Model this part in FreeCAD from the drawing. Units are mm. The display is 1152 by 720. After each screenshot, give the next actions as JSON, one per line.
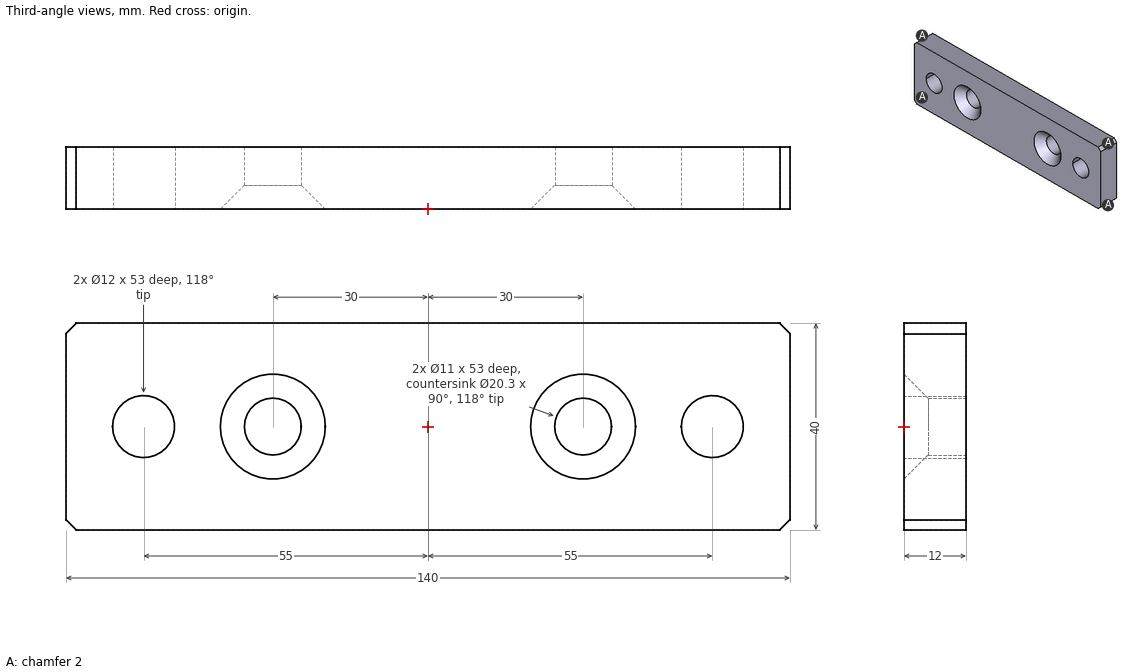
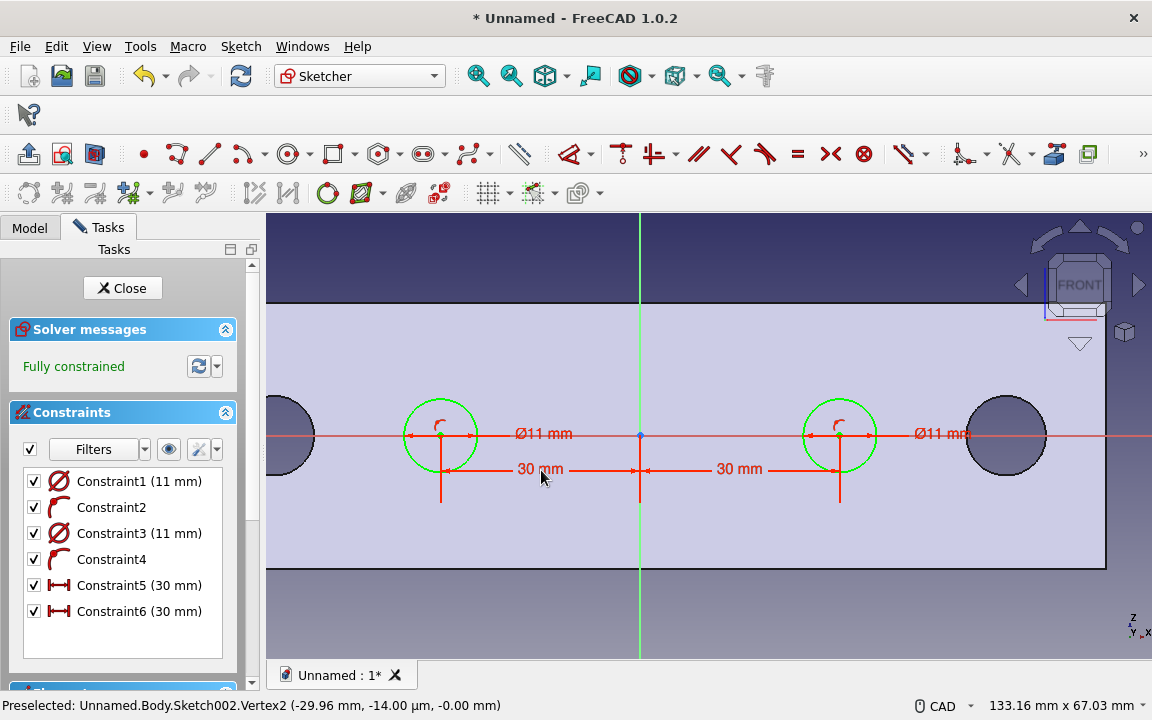
{"action": "left_click", "coordinate": [123, 288]}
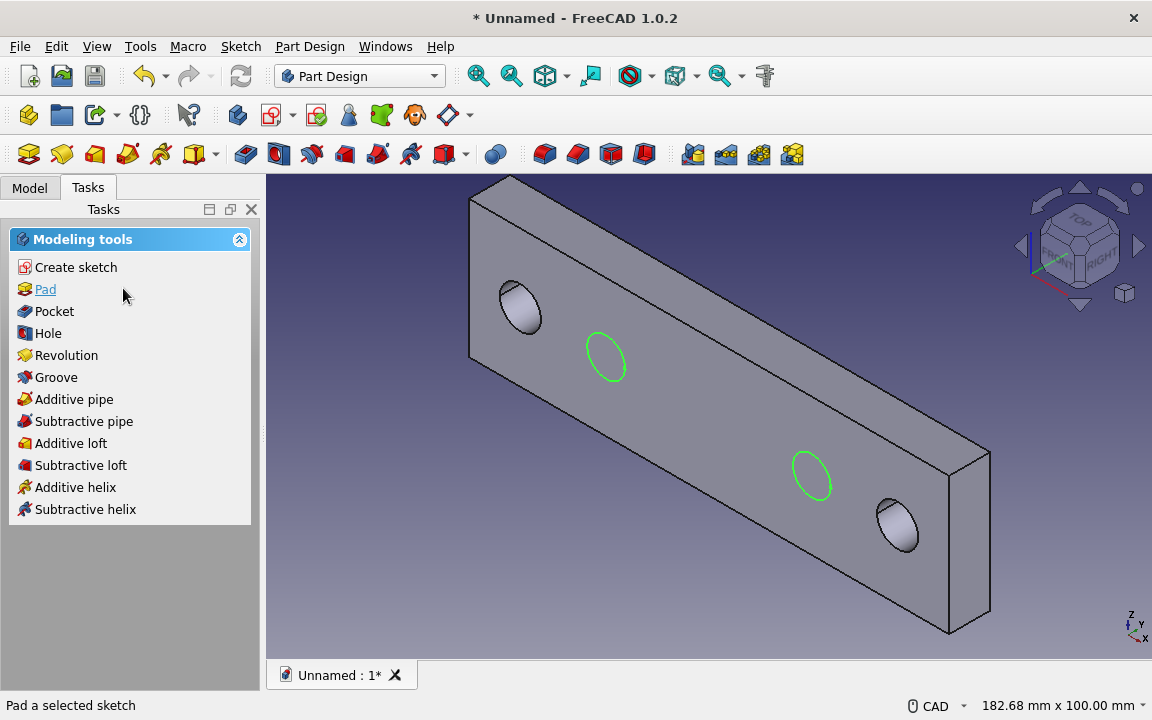
{"action": "left_click", "coordinate": [279, 154]}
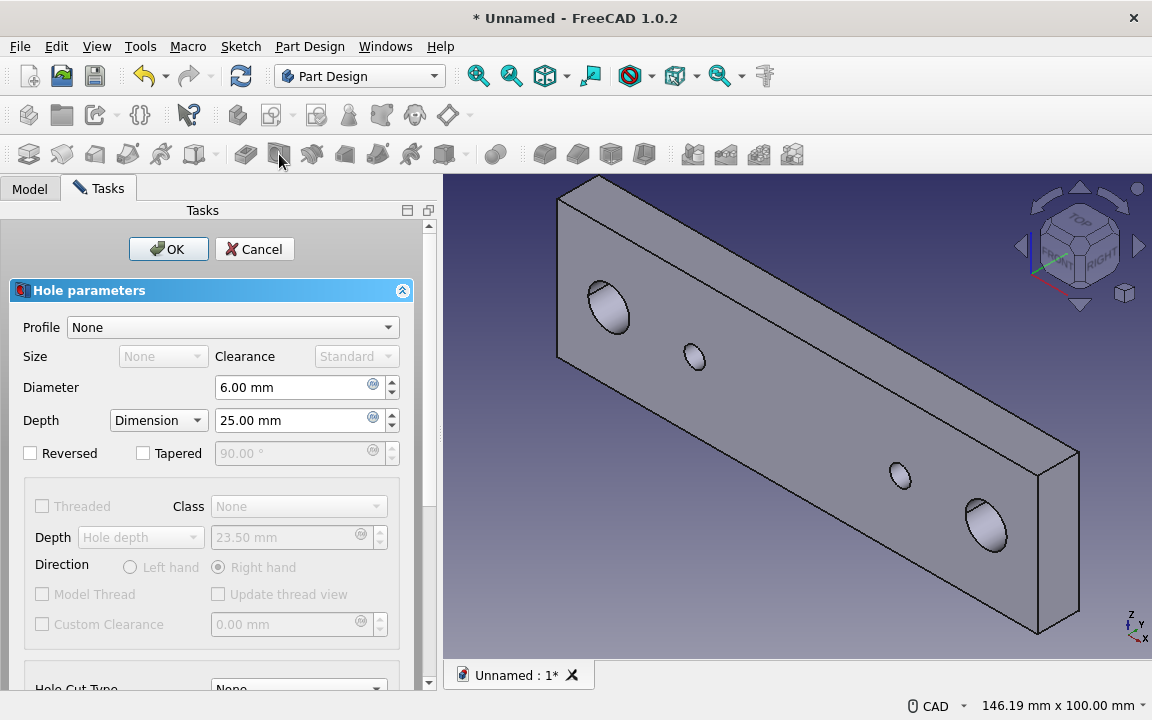
{"action": "triple_click", "coordinate": [300, 388]}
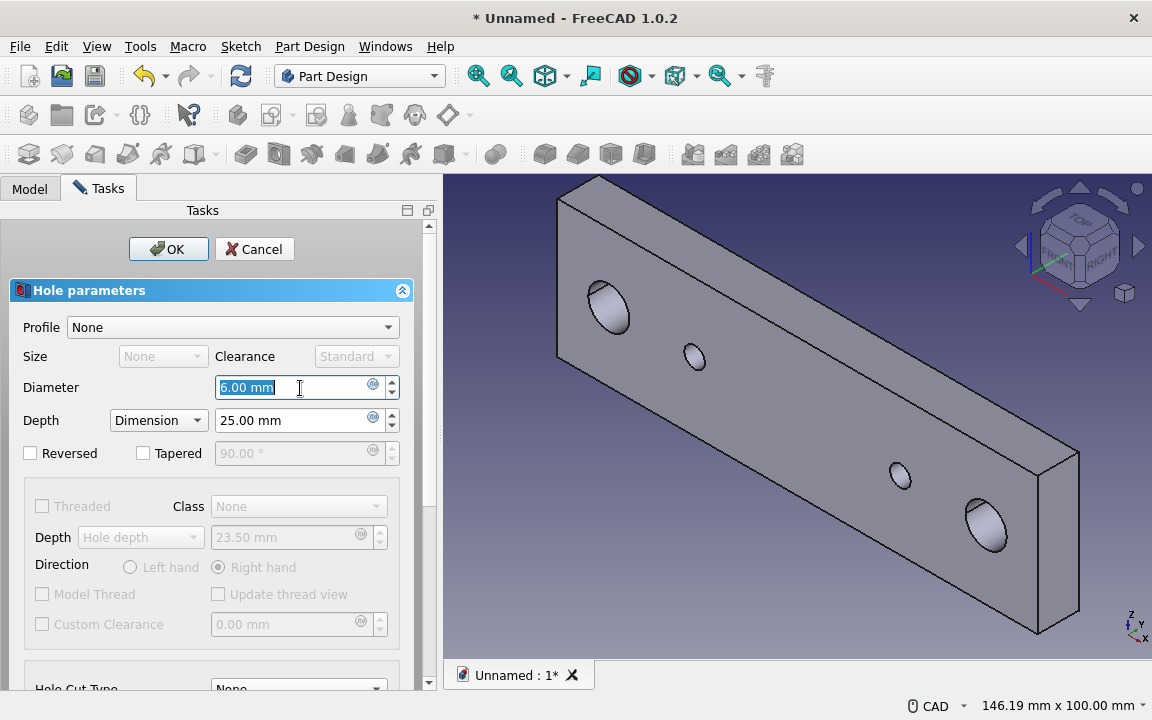
{"action": "type", "text": "11"}
{"action": "key", "text": "Tab"}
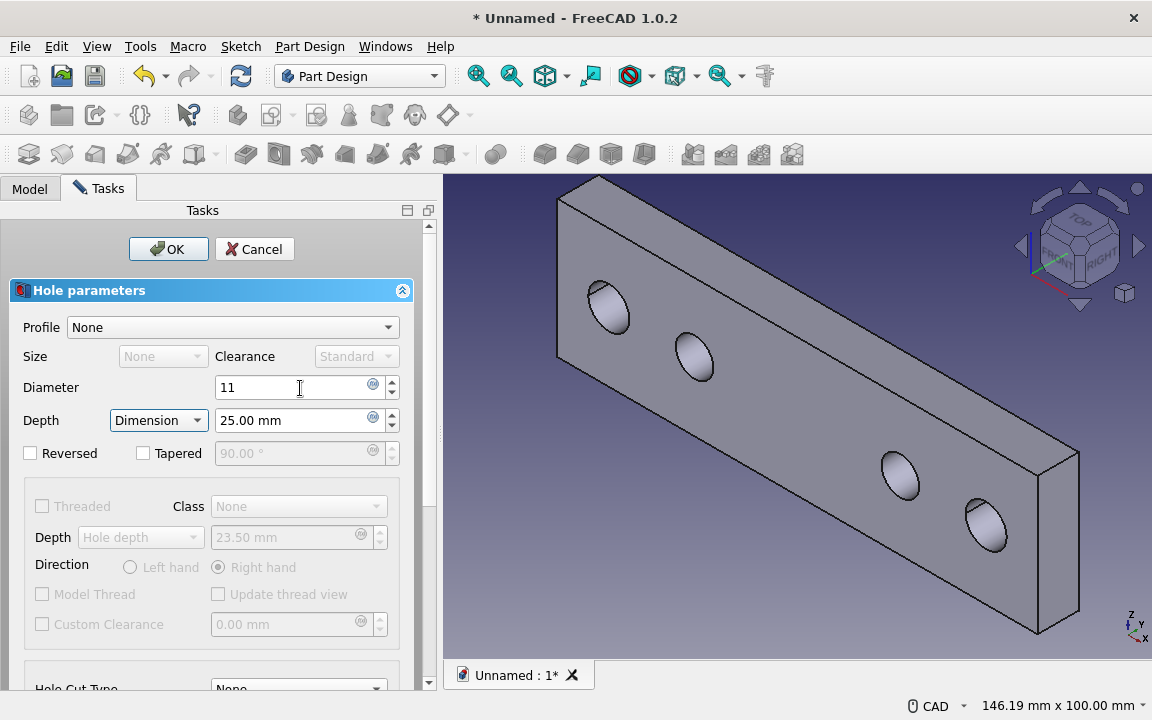
{"action": "triple_click", "coordinate": [300, 420]}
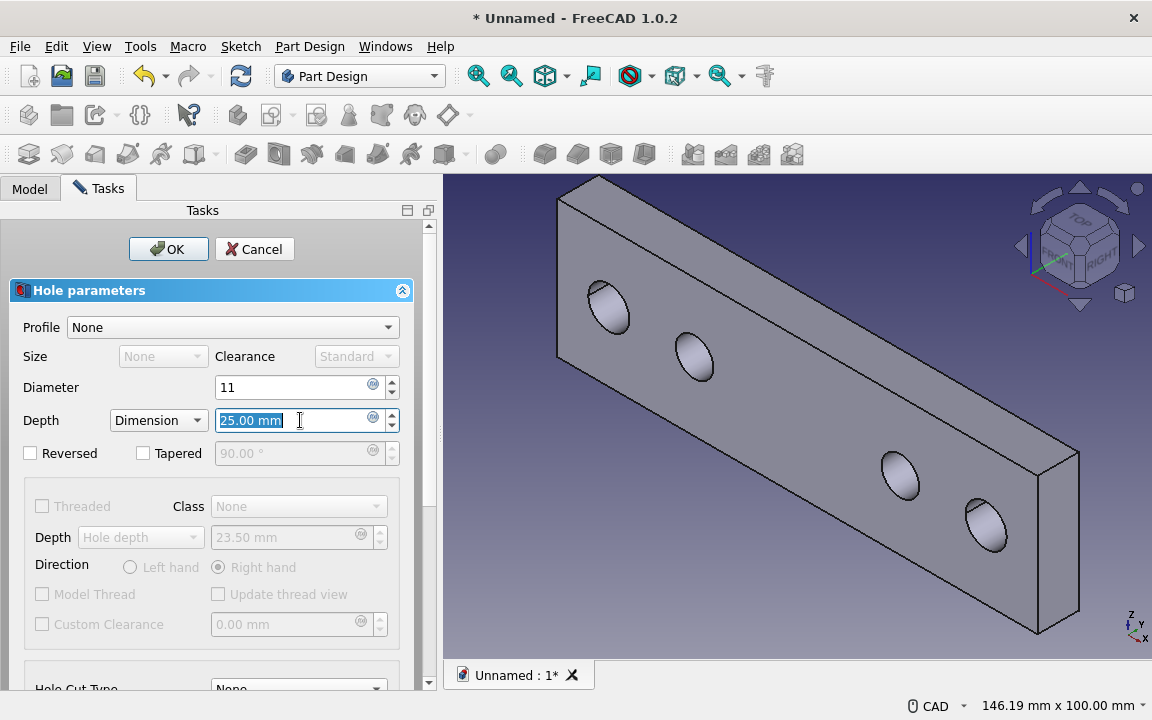
{"action": "type", "text": "53"}
{"action": "key", "text": "Tab"}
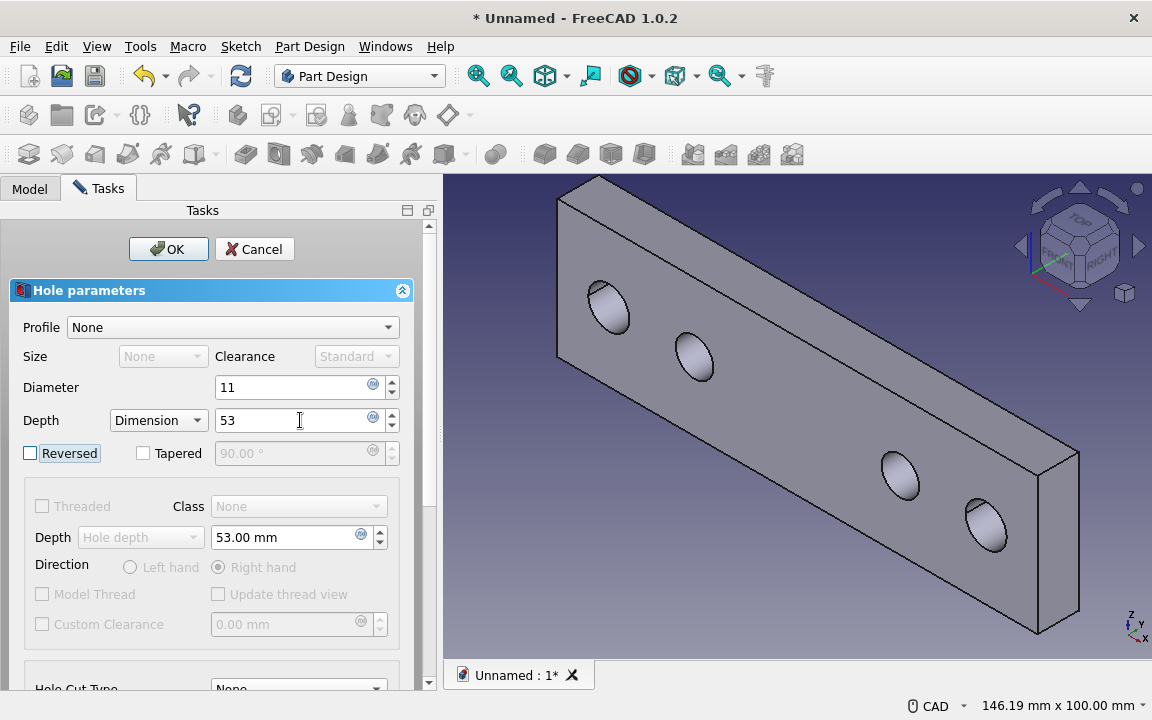
{"action": "scroll", "coordinate": [429, 455], "scroll_direction": "down", "scroll_amount": 2}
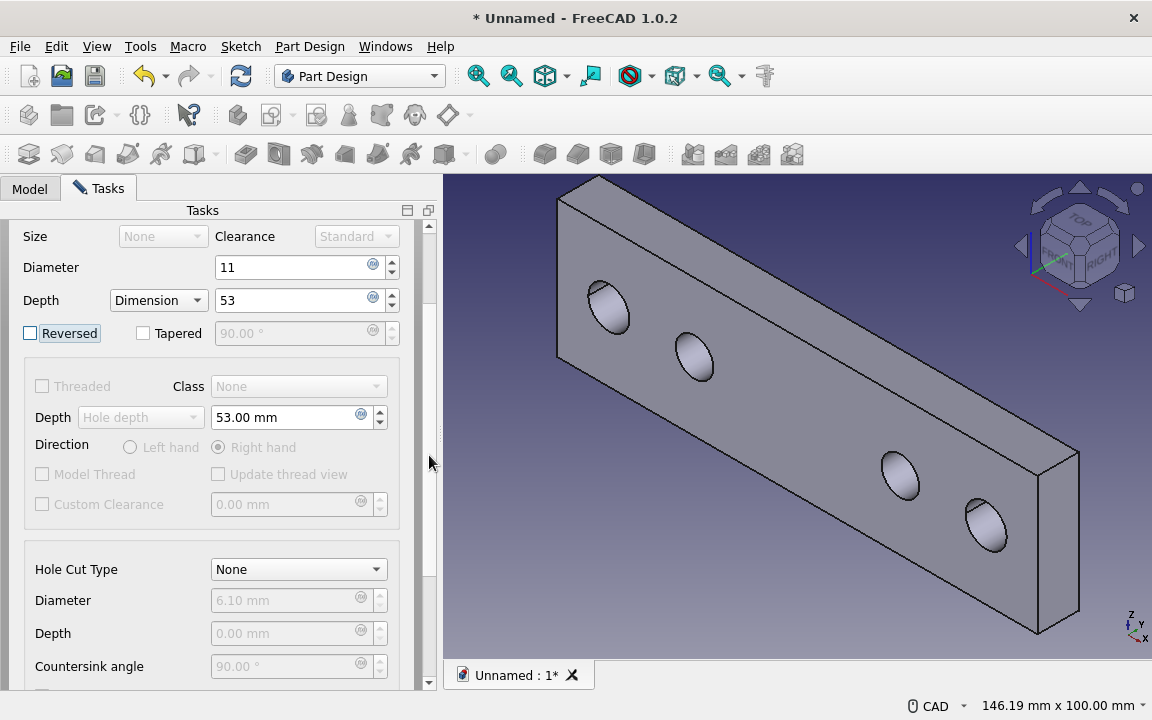
{"action": "left_click", "coordinate": [300, 570]}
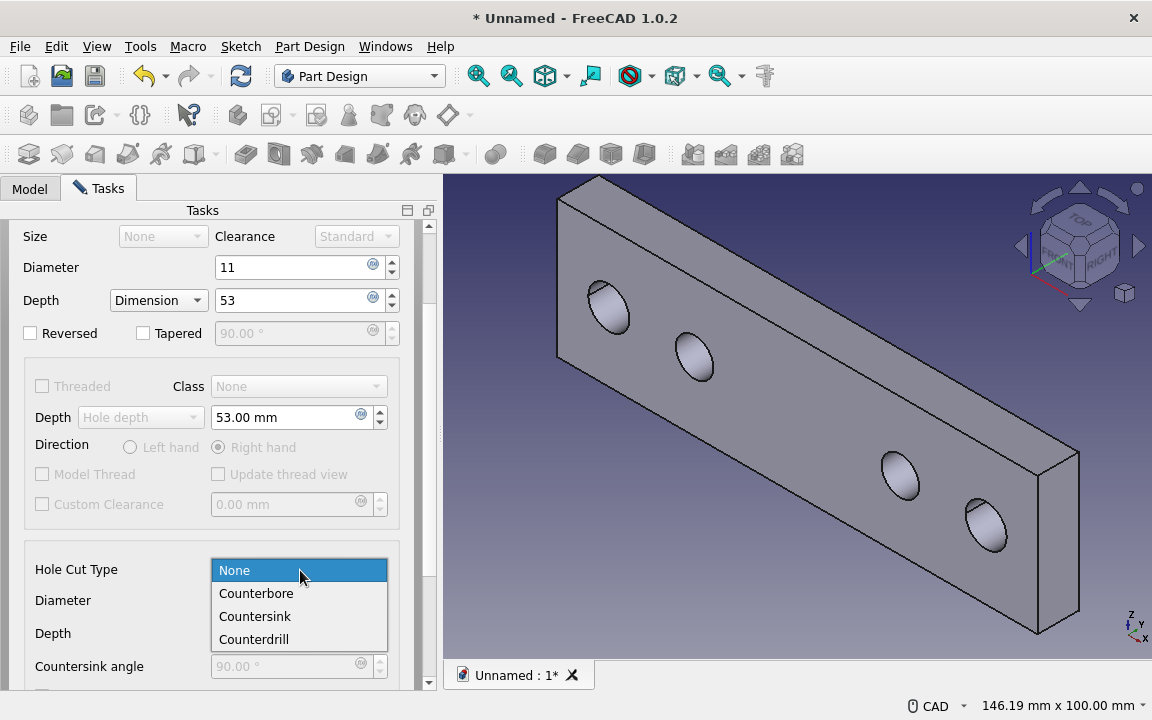
{"action": "left_click", "coordinate": [298, 616]}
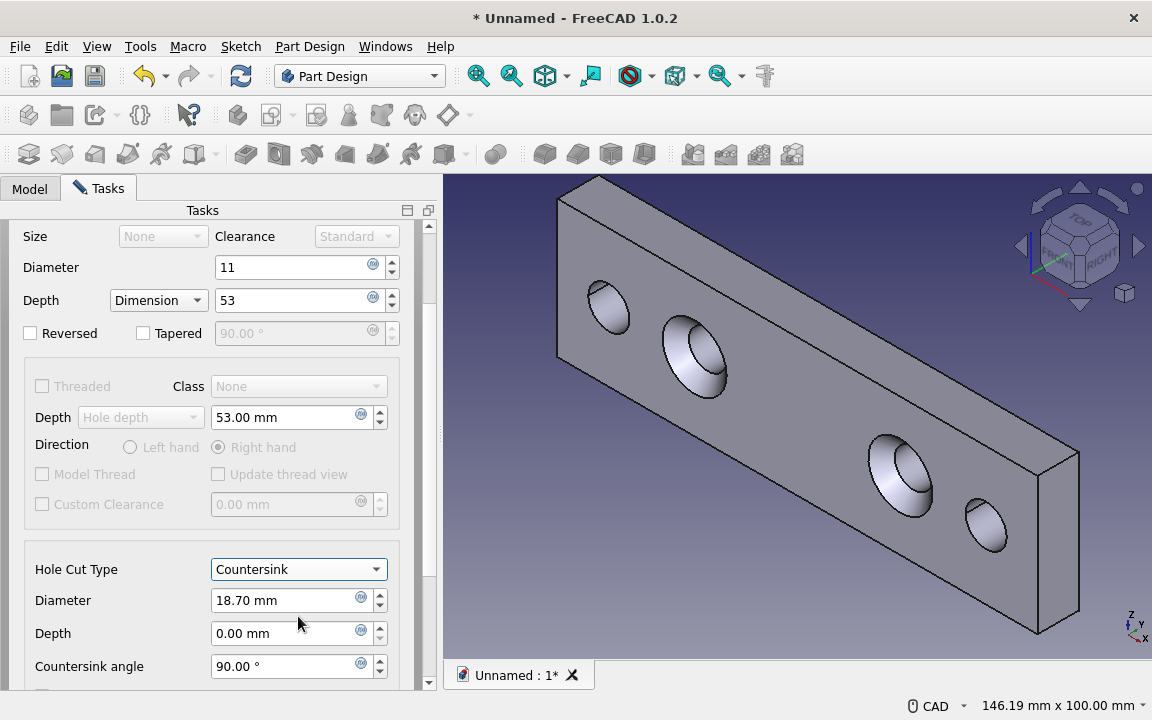
{"action": "triple_click", "coordinate": [292, 600]}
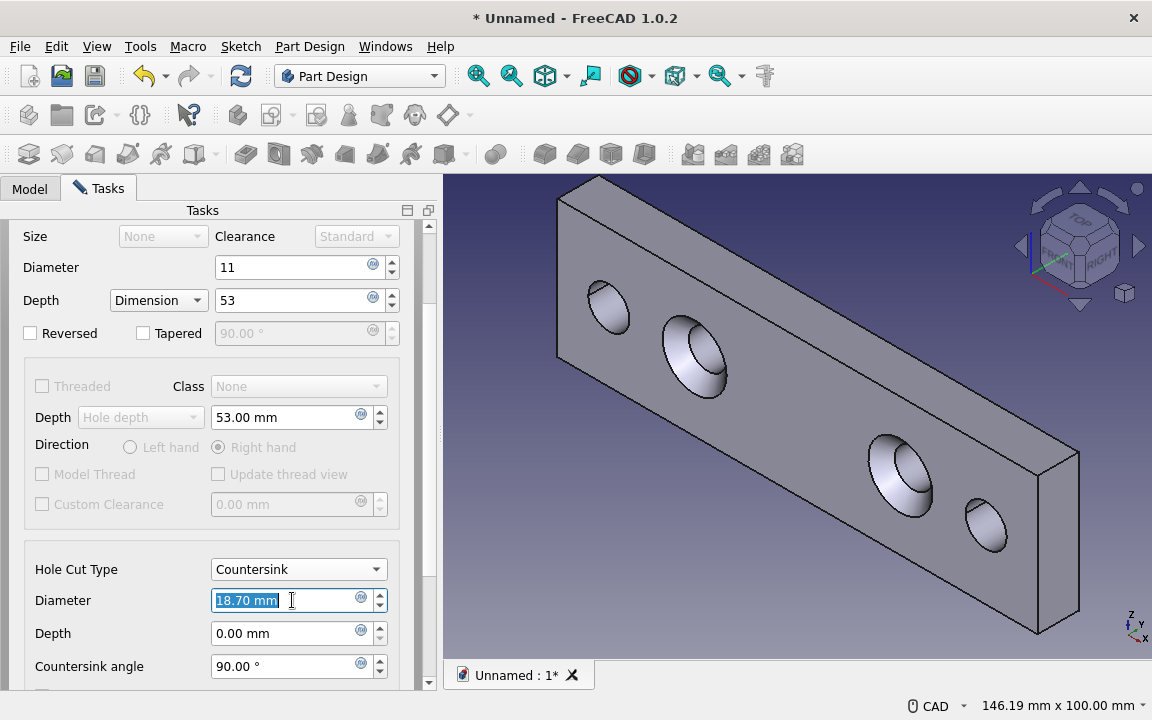
{"action": "type", "text": "20.3"}
{"action": "key", "text": "Tab"}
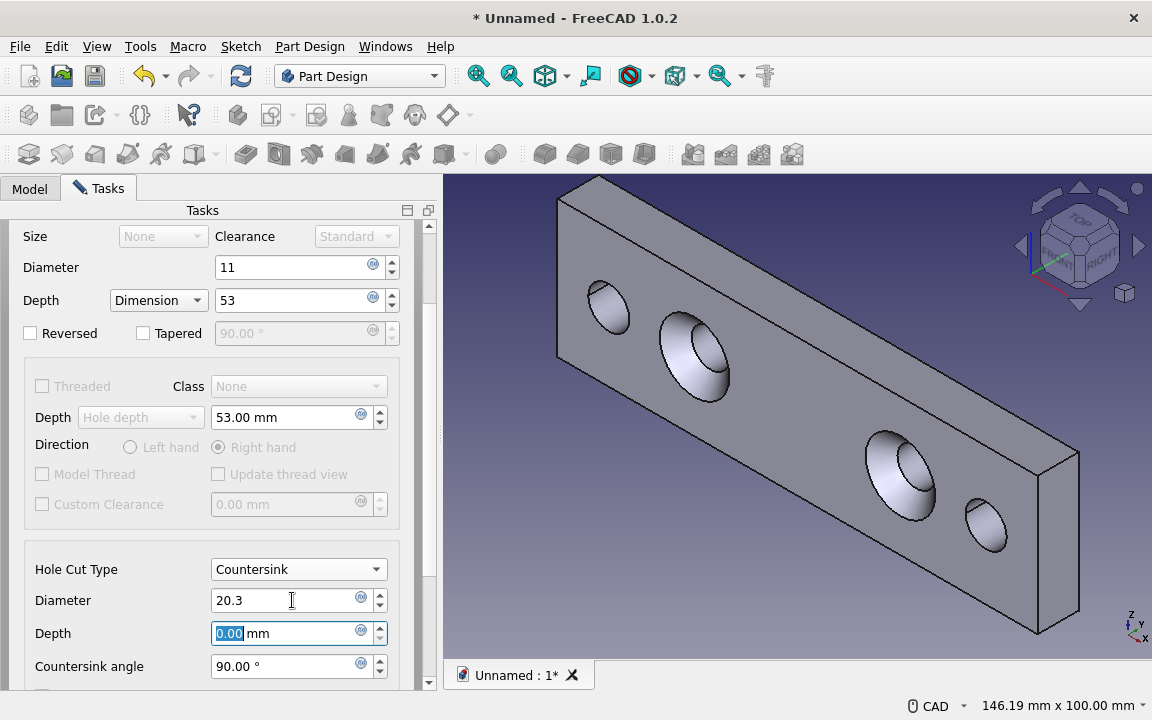
{"action": "scroll", "coordinate": [429, 455], "scroll_direction": "up", "scroll_amount": 3}